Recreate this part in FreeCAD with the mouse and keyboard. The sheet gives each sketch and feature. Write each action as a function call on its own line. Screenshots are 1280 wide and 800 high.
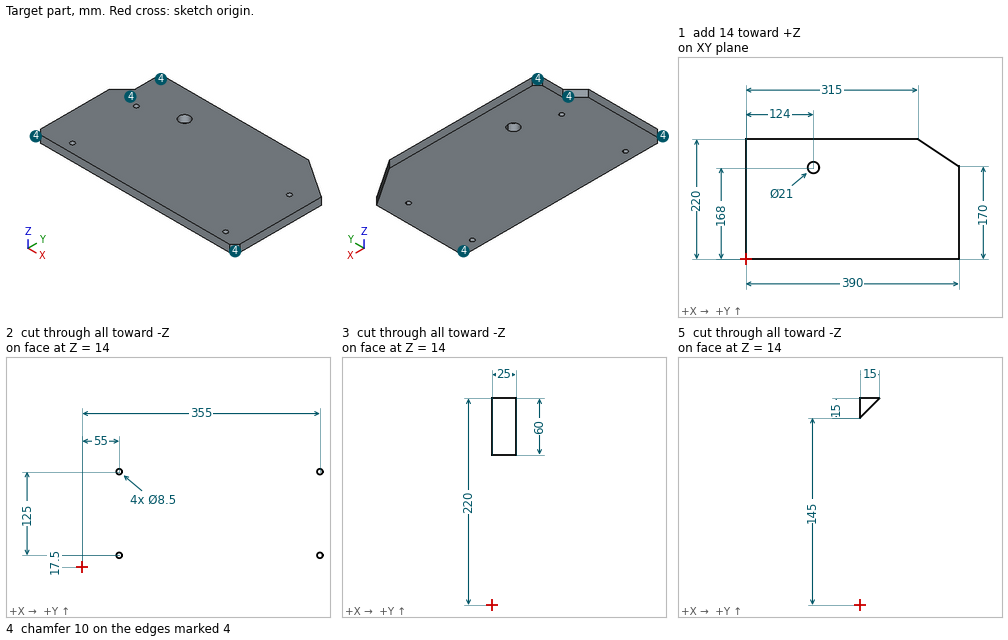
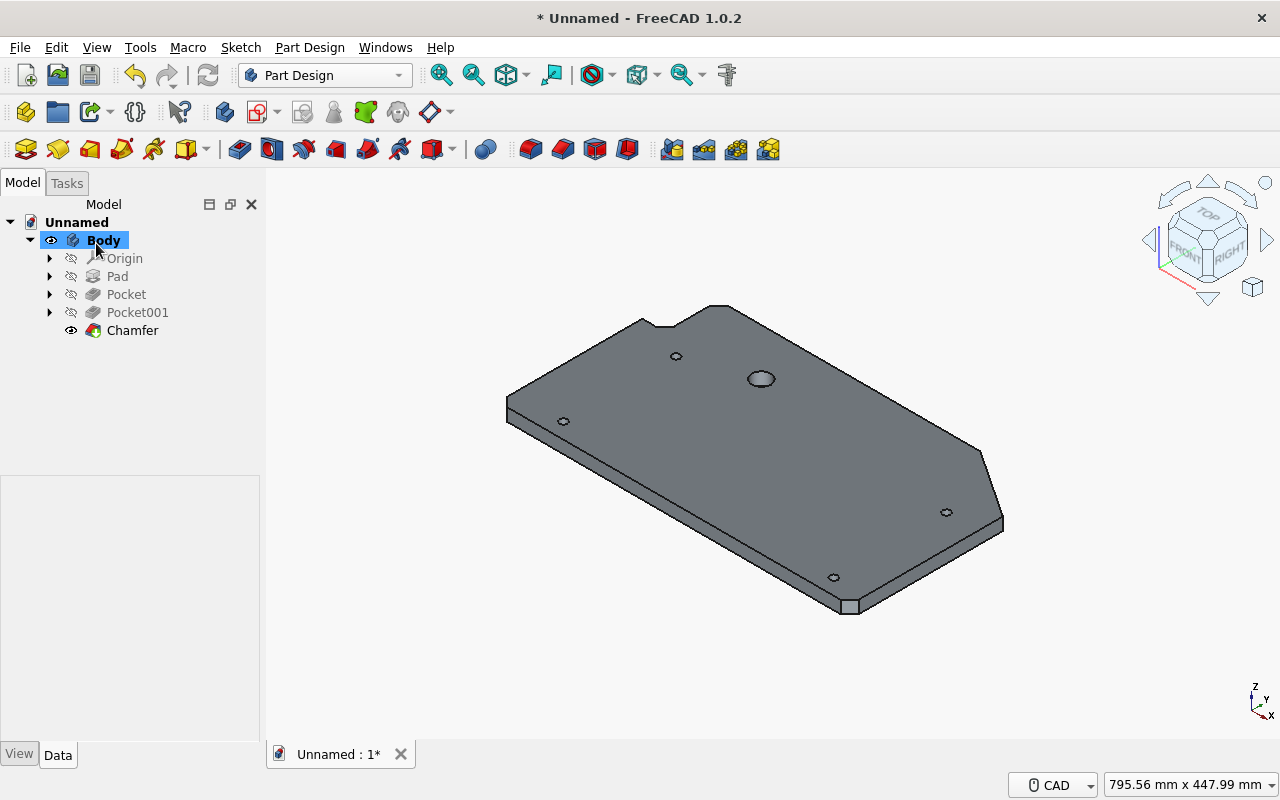
click(823, 474)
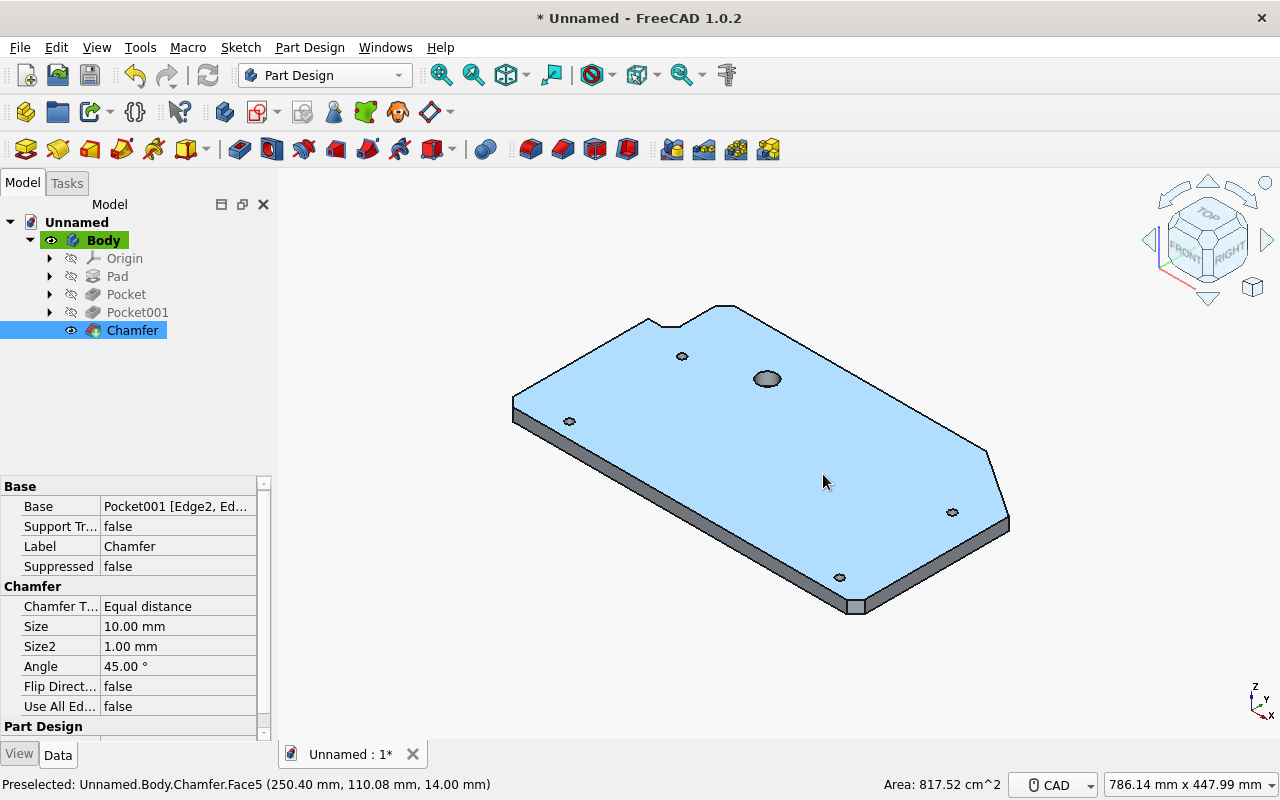
click(258, 112)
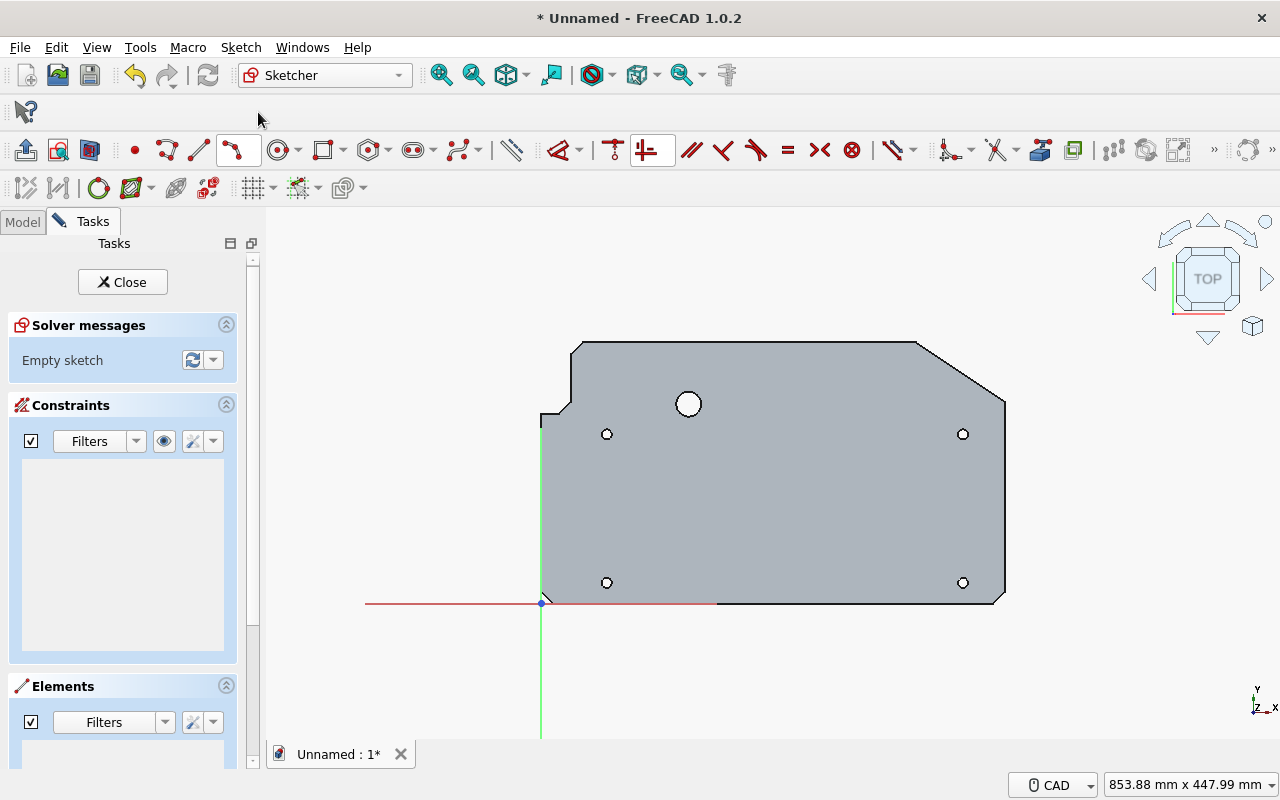
scroll(542, 420, up, 15)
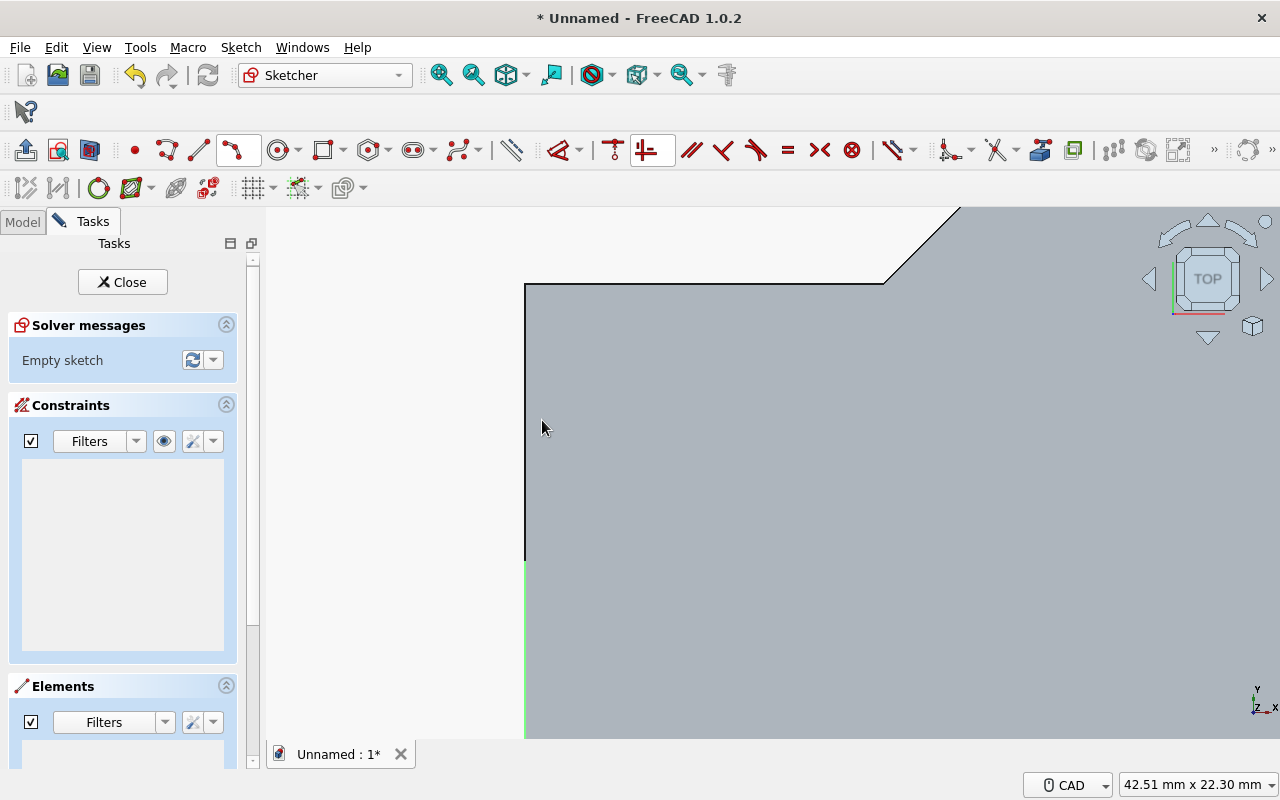
click(168, 150)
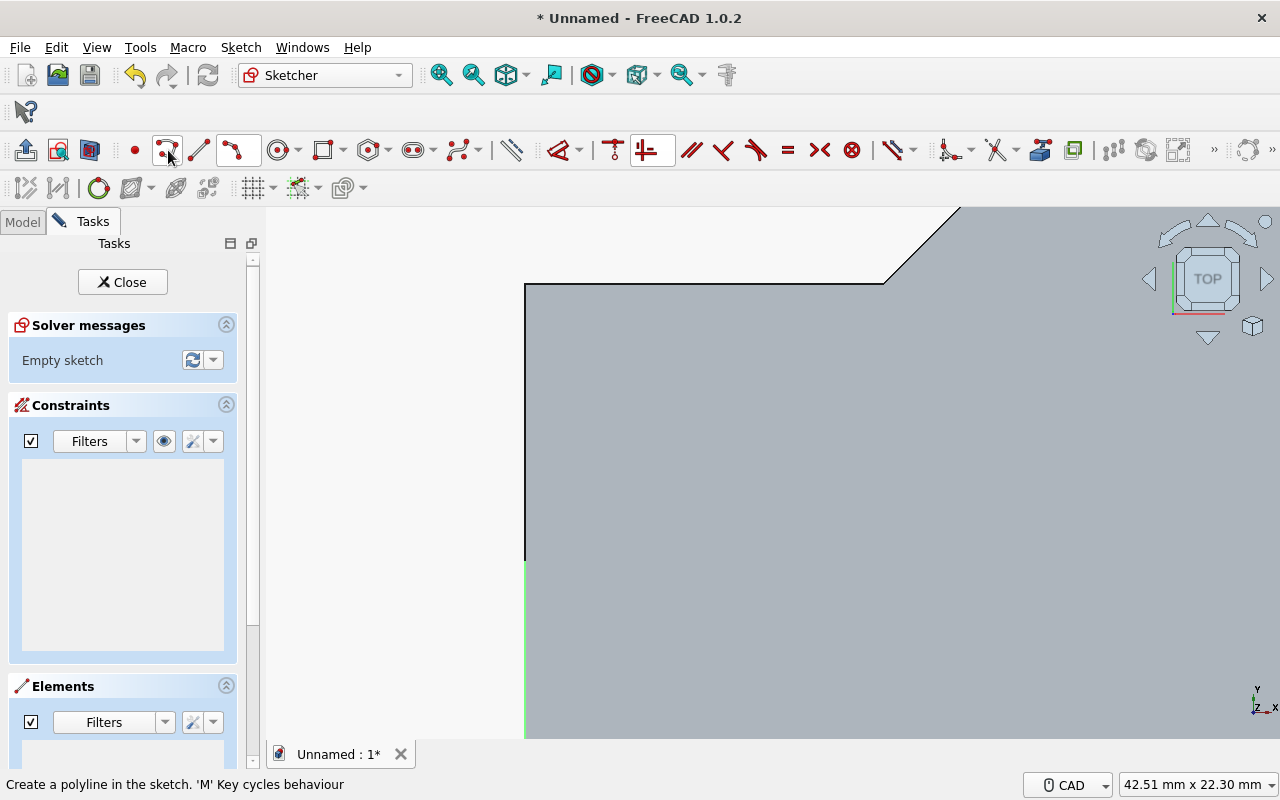
click(525, 642)
click(883, 284)
click(534, 284)
click(525, 643)
key(Escape)
key(Escape)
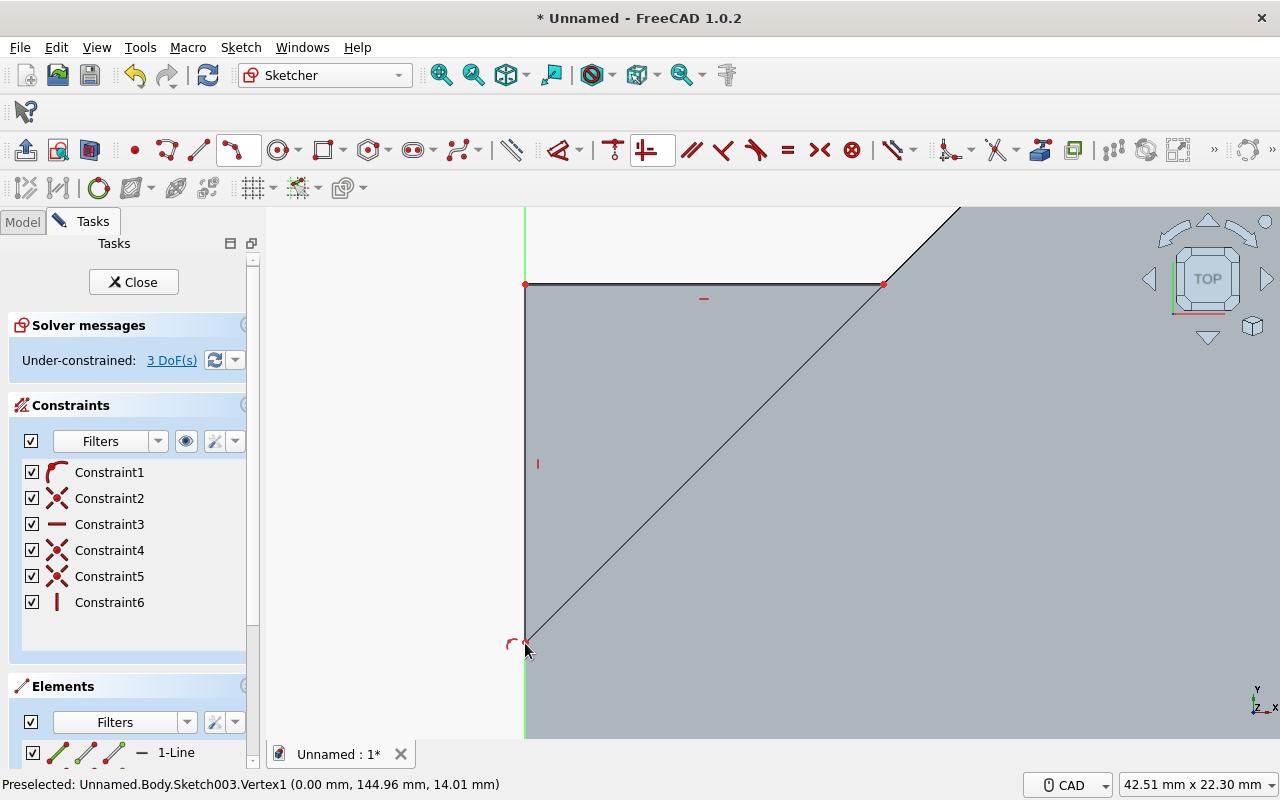
key(d)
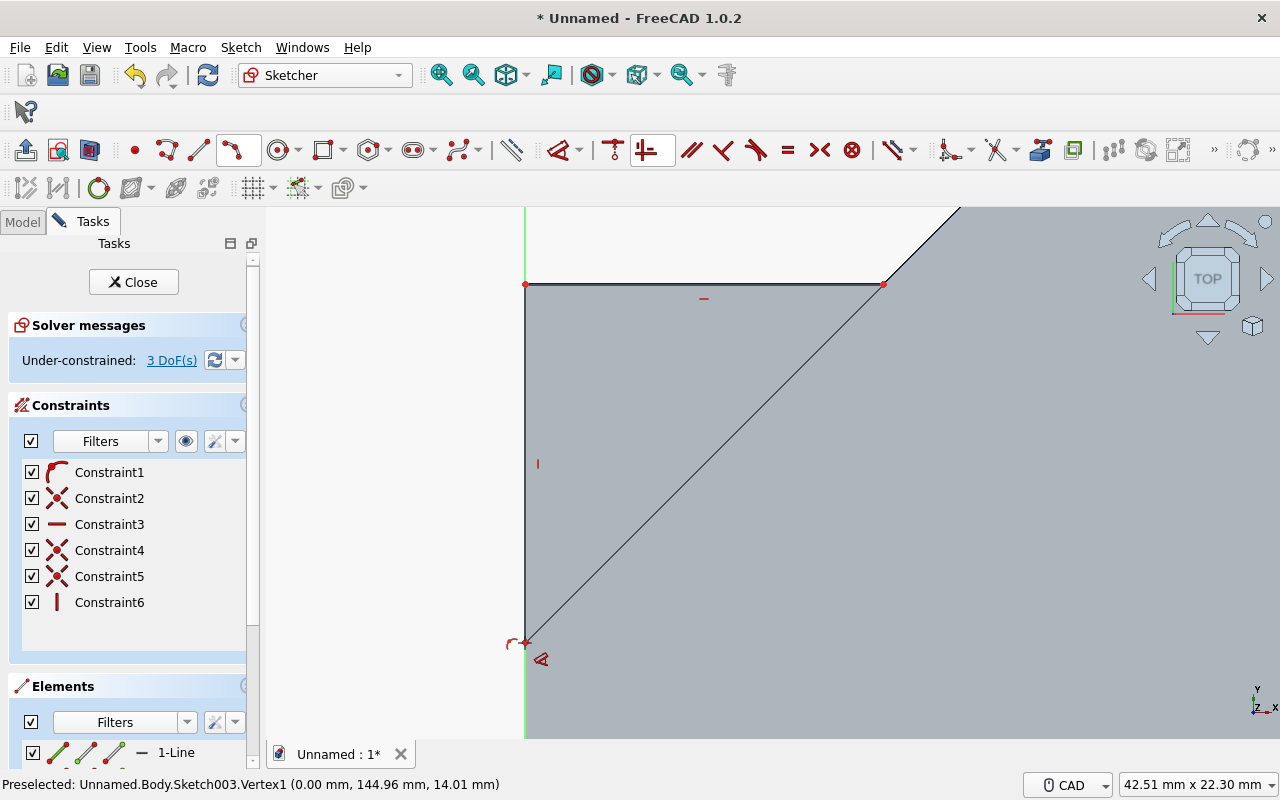
click(776, 285)
click(704, 251)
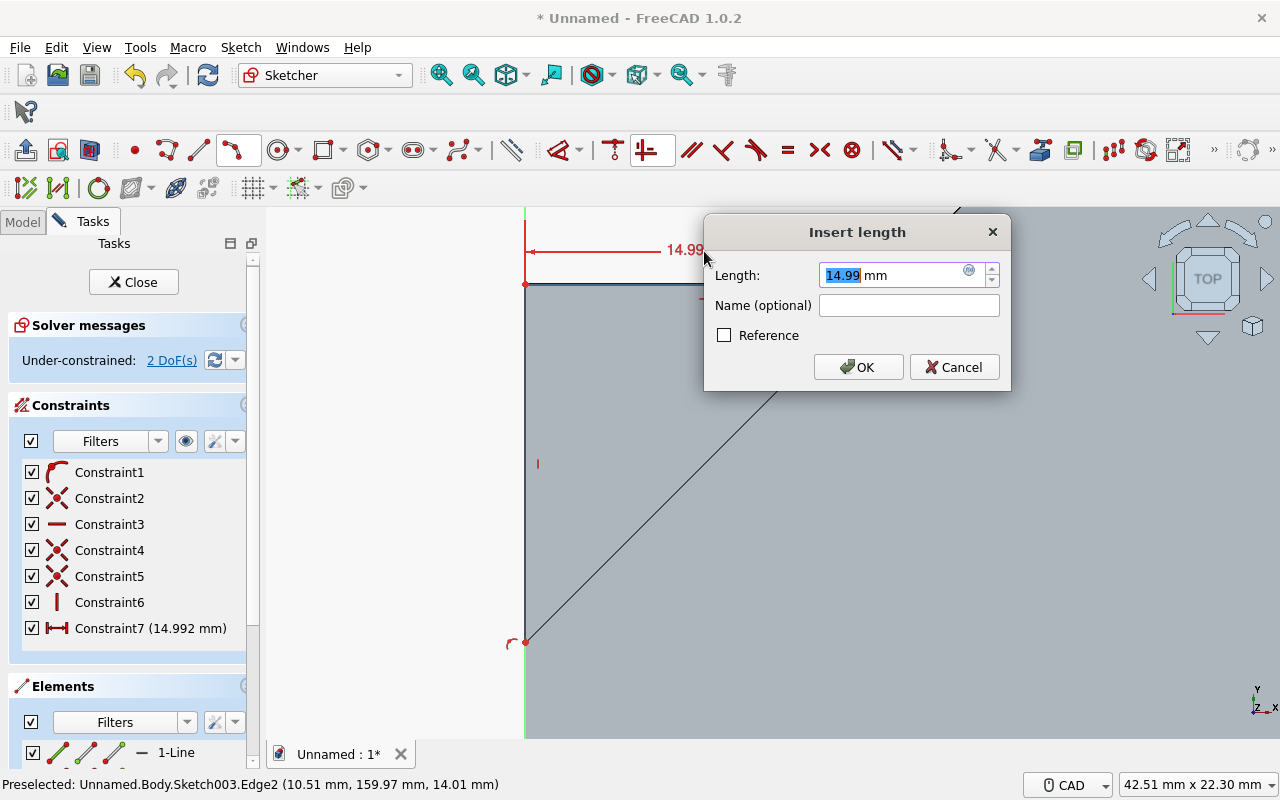
text(15)
key(Return)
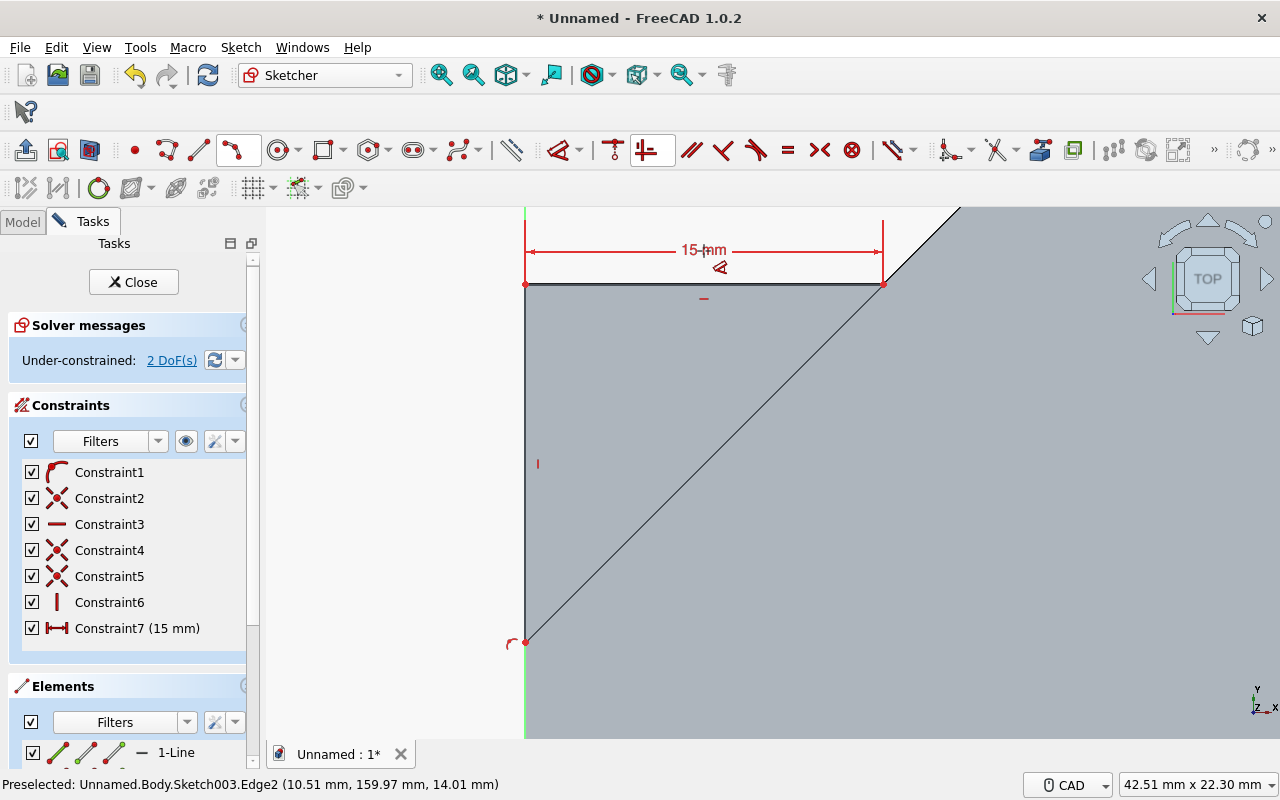
click(525, 392)
click(491, 464)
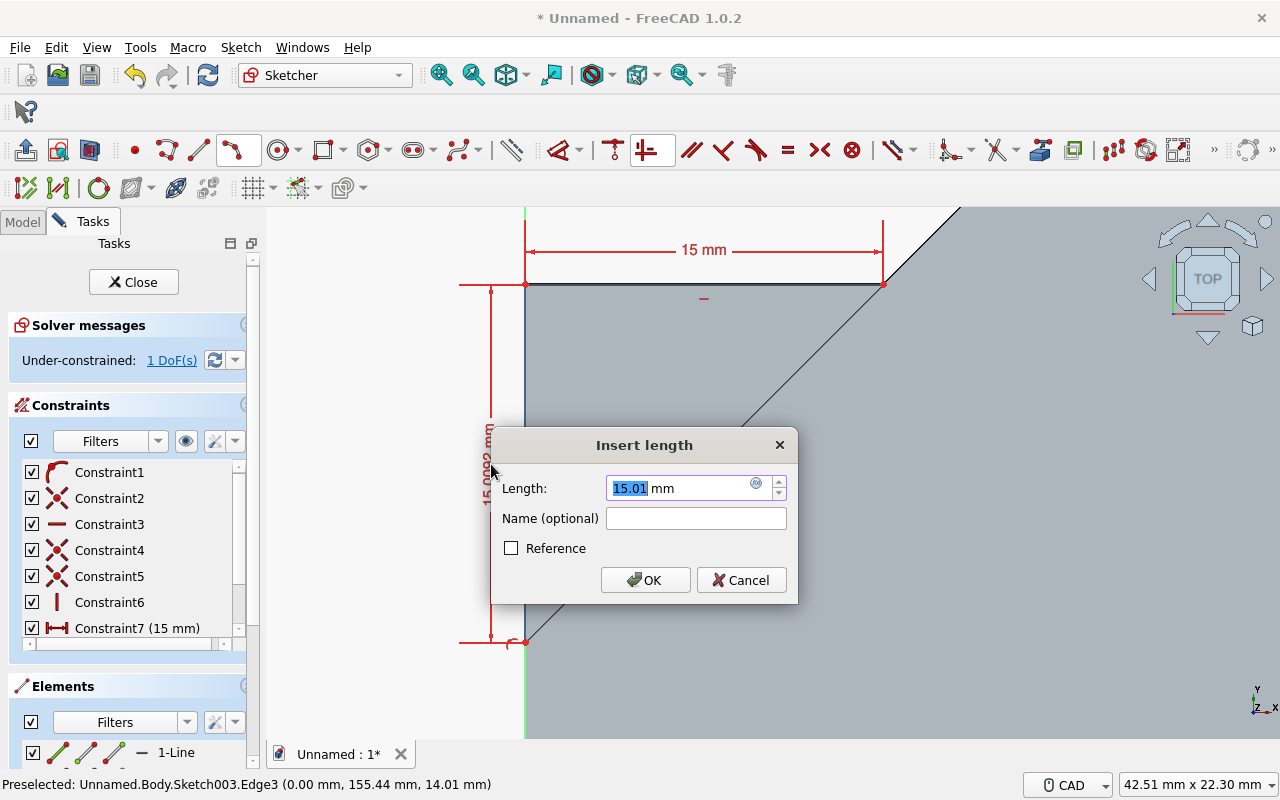
text(15)
key(Return)